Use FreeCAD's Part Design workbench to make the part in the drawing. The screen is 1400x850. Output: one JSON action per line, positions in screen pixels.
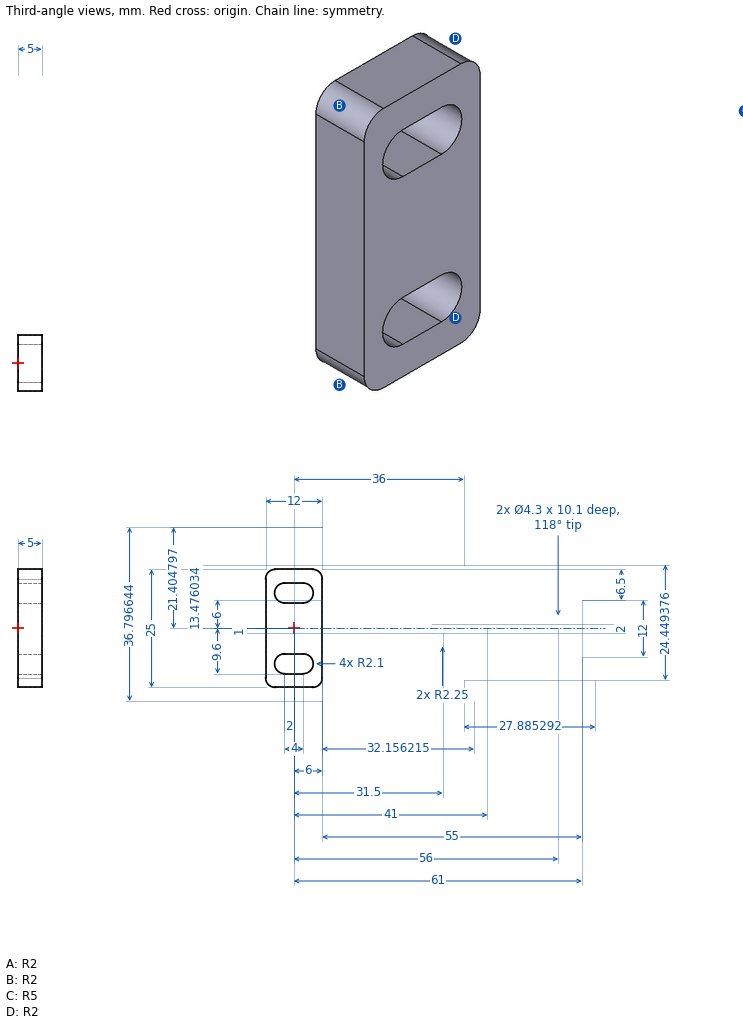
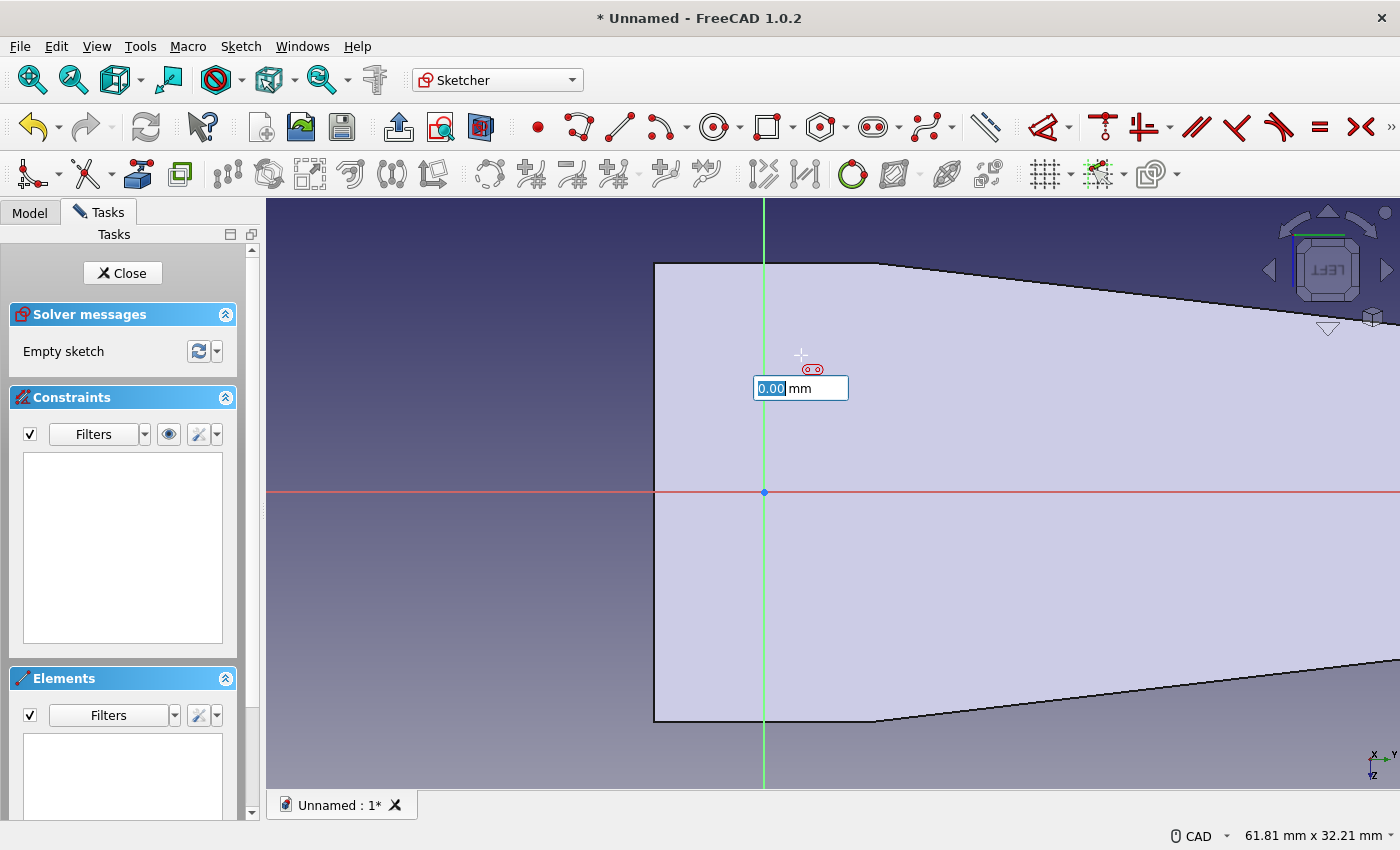
{"action": "scroll", "coordinate": [753, 393], "scroll_direction": "up", "scroll_amount": 2}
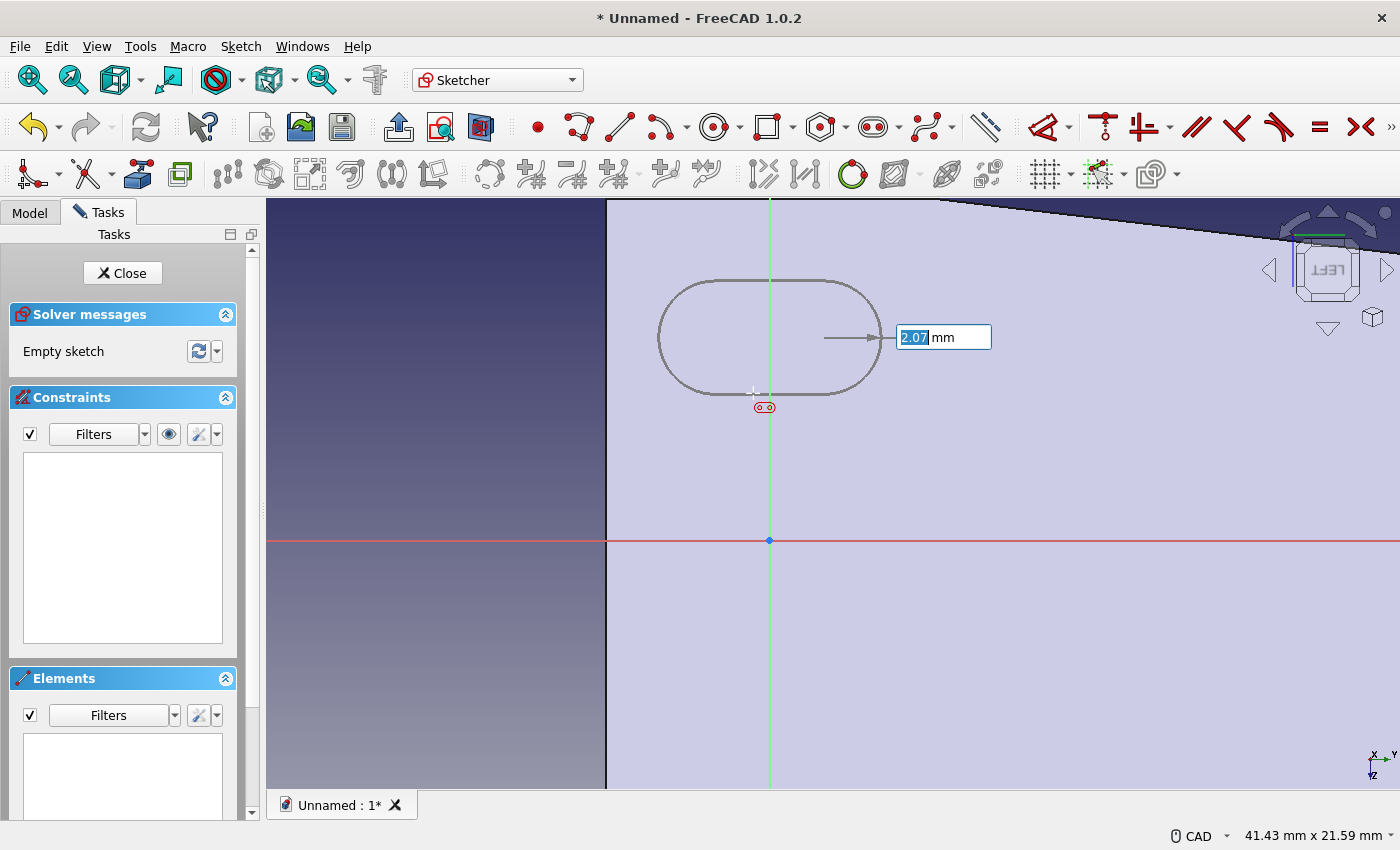
{"action": "left_click", "coordinate": [754, 393]}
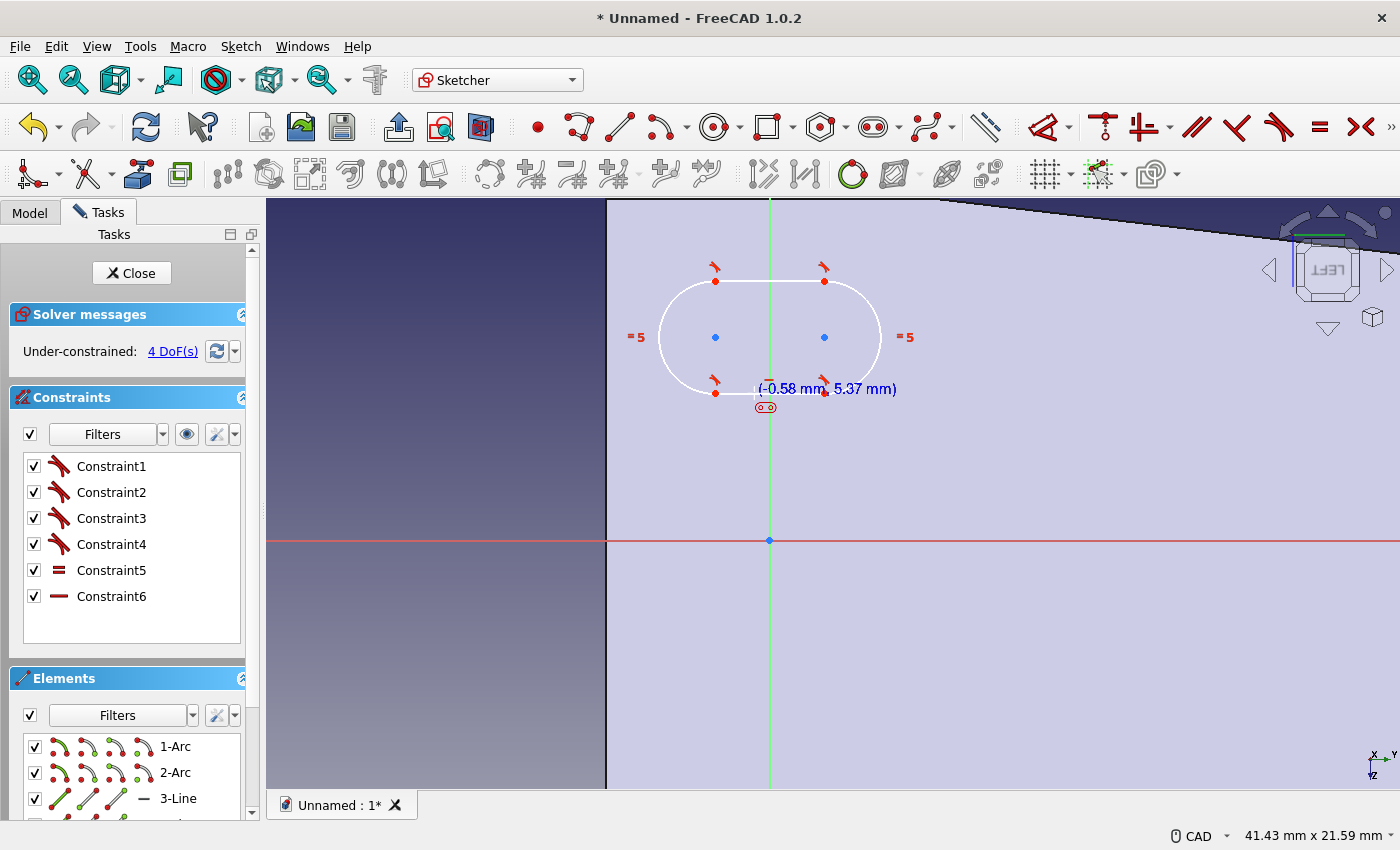
{"action": "left_click", "coordinate": [715, 746]}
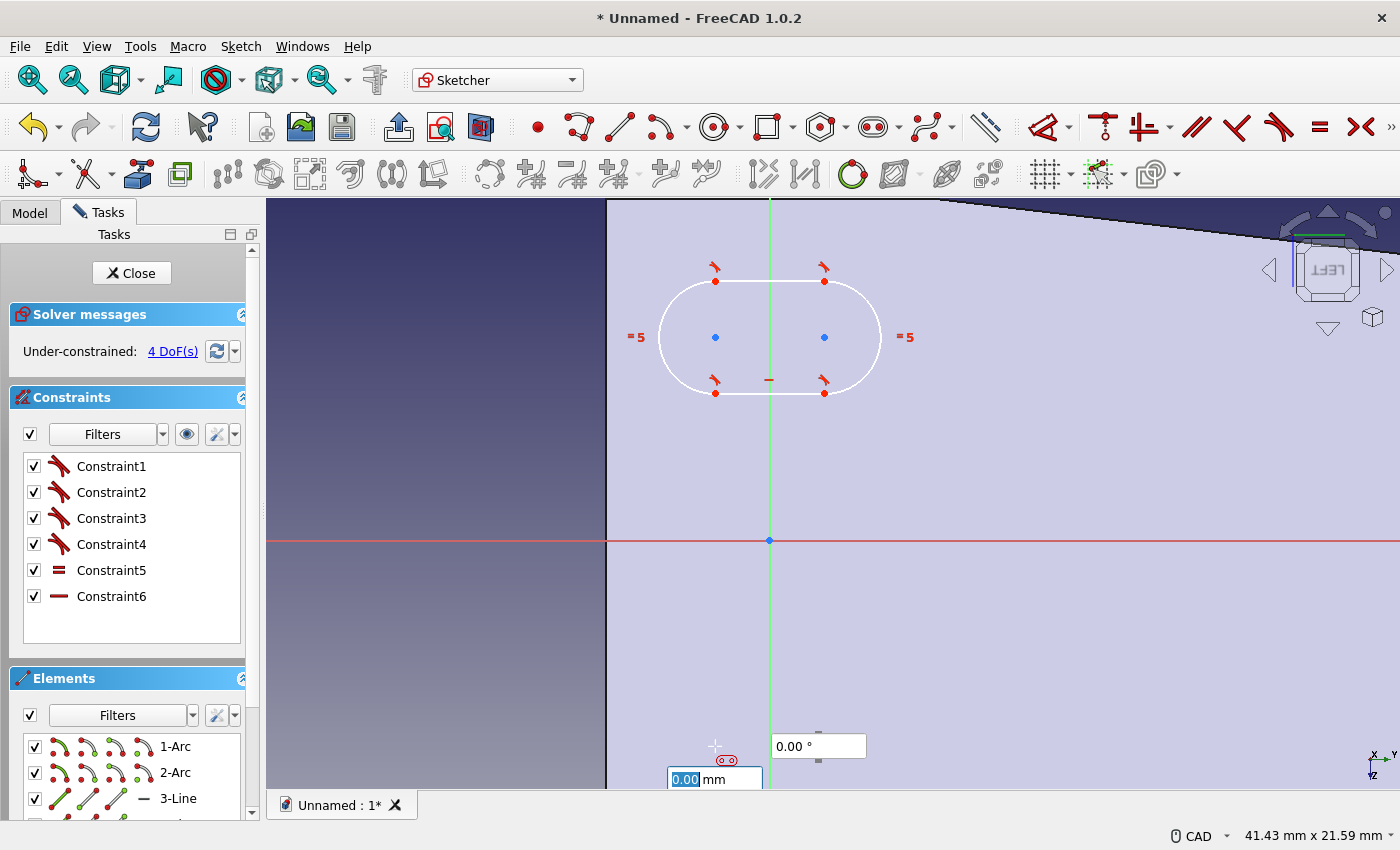
{"action": "left_click", "coordinate": [825, 746]}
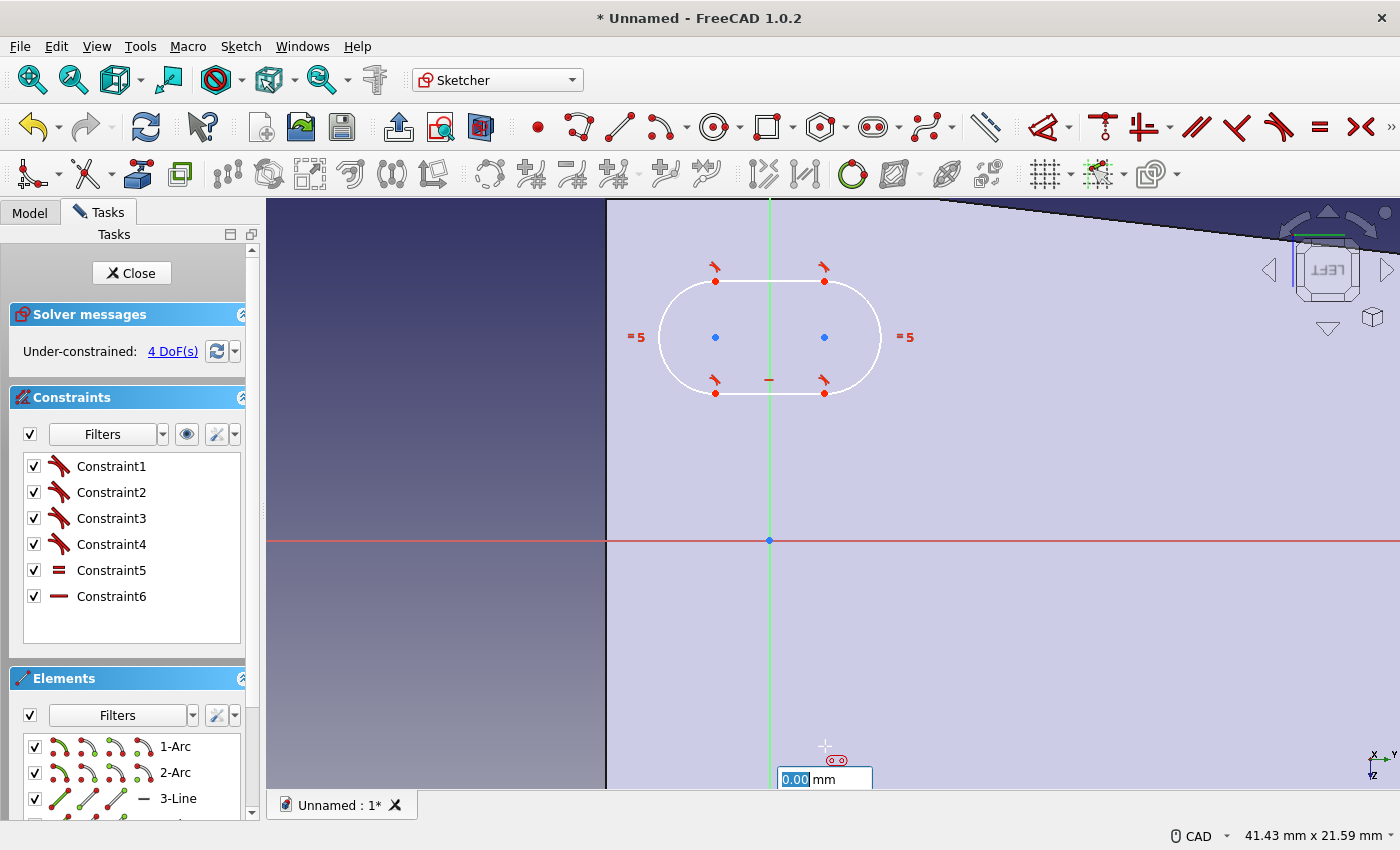
{"action": "left_click", "coordinate": [786, 689]}
{"action": "key", "text": "Escape"}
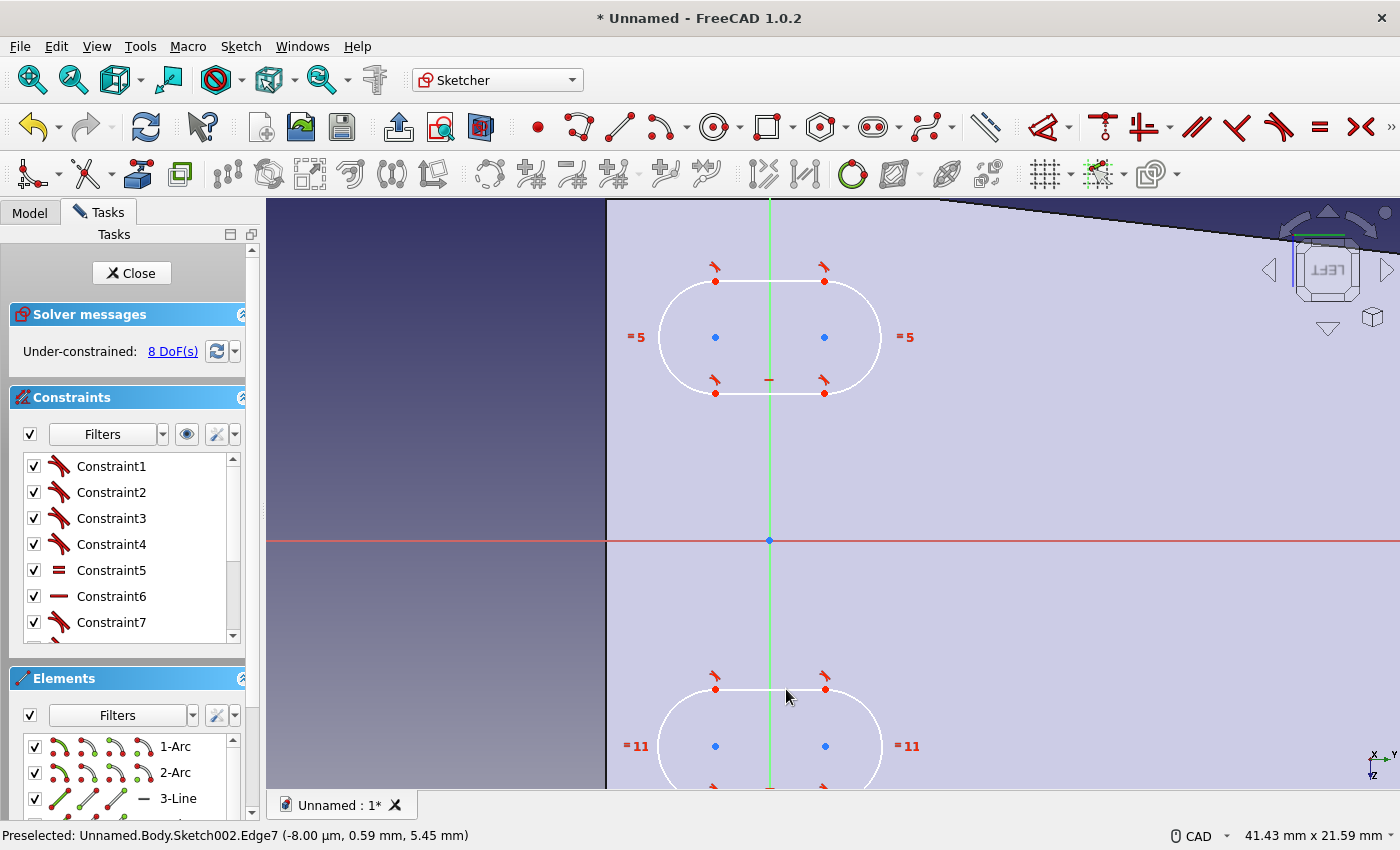
{"action": "left_click", "coordinate": [670, 305]}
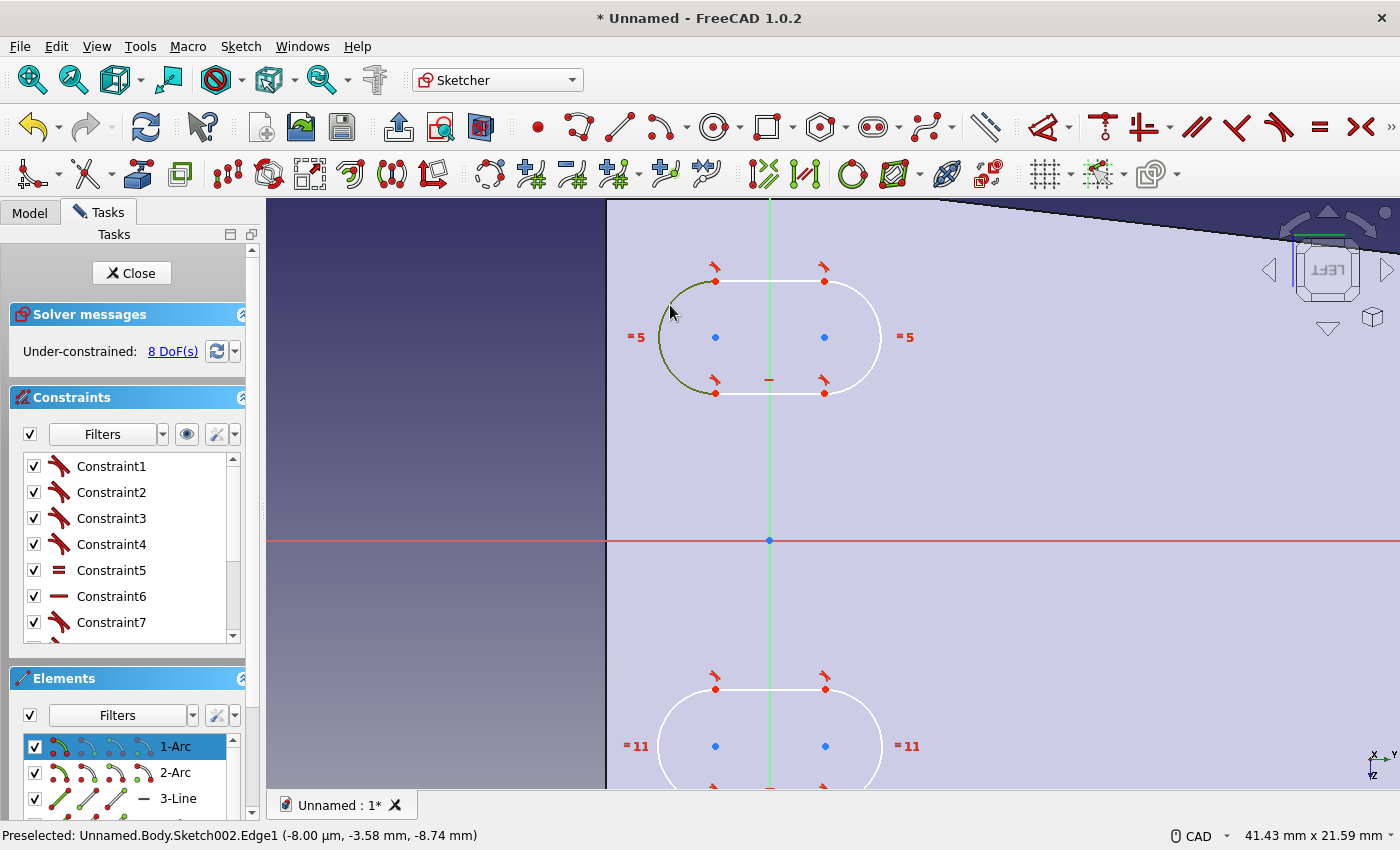
{"action": "left_click", "coordinate": [669, 713]}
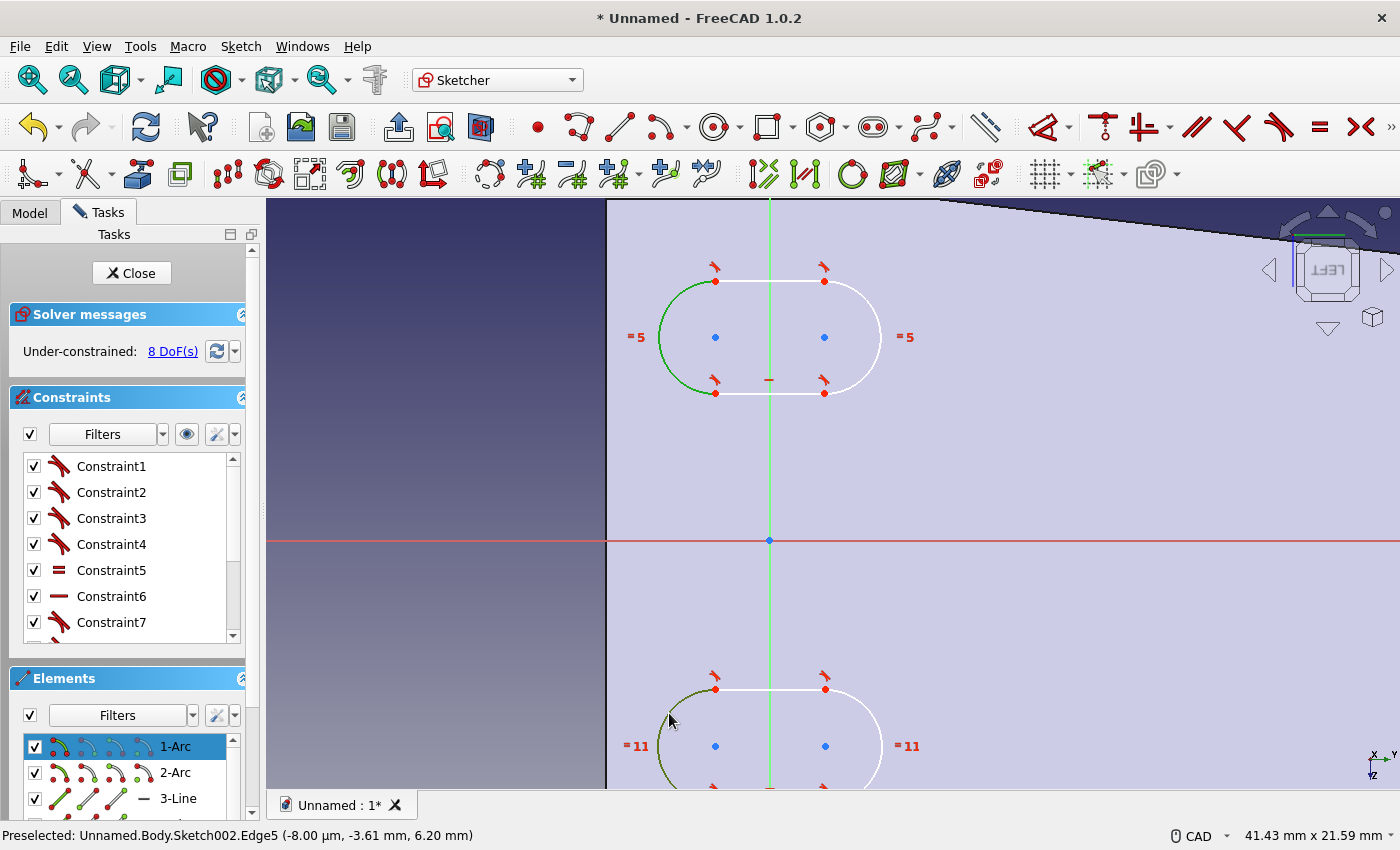
{"action": "left_click", "coordinate": [1320, 128]}